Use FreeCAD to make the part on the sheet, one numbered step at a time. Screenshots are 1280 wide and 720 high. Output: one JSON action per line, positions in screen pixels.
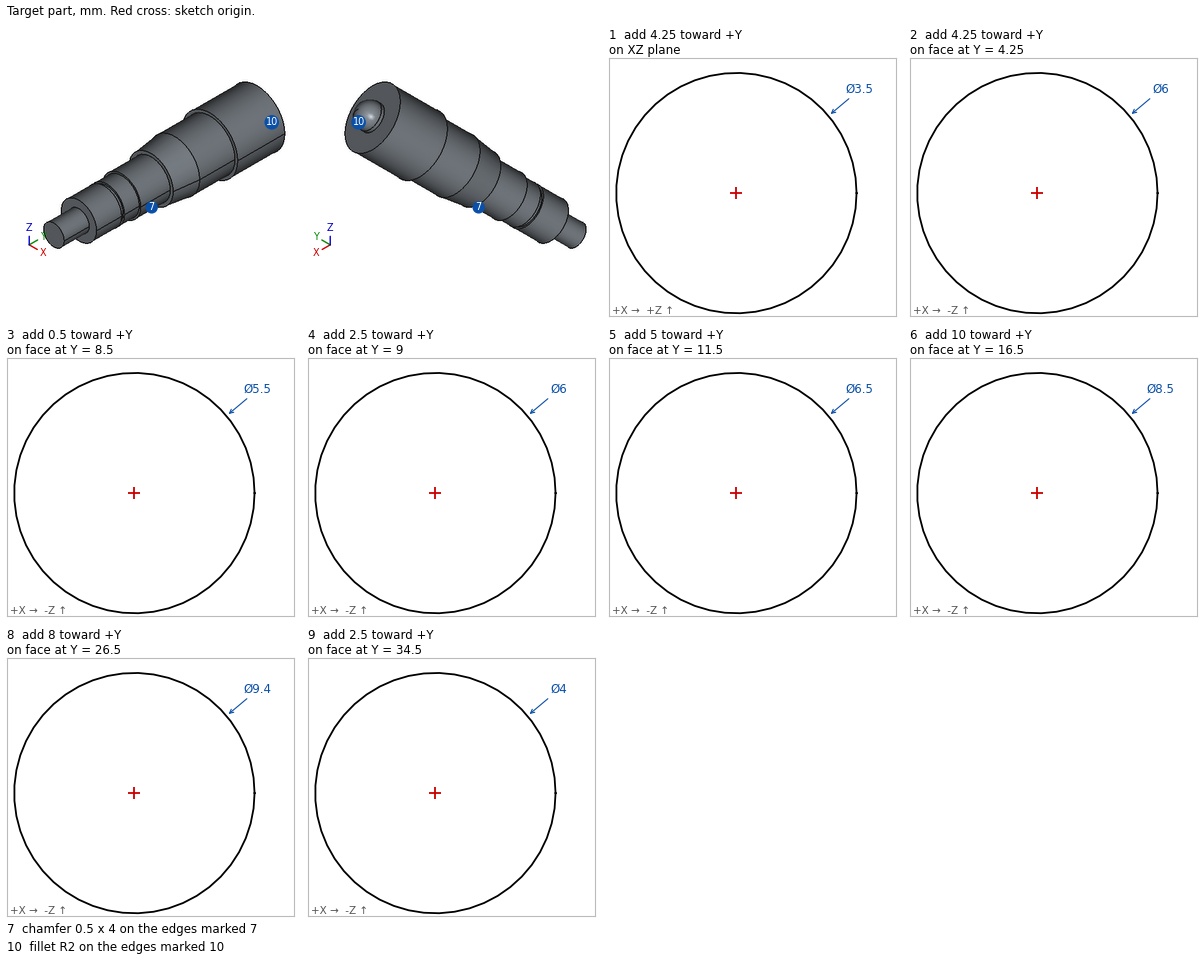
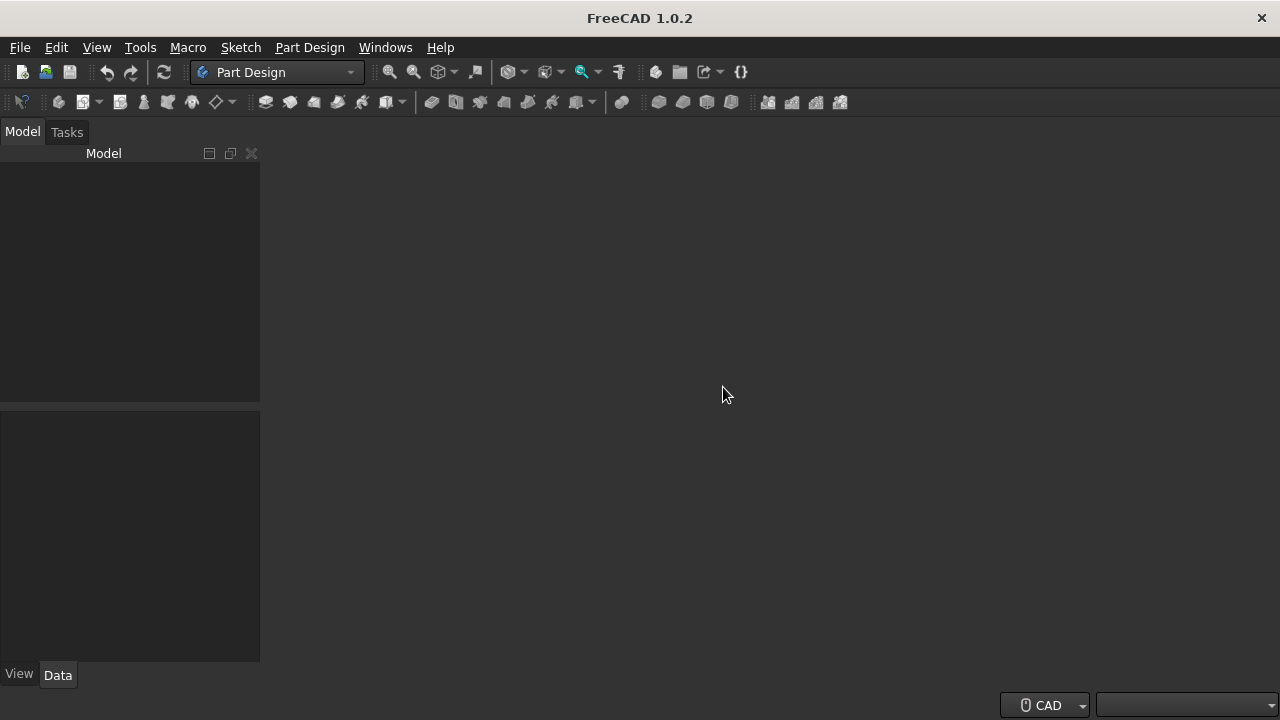
{"action": "key", "text": "ctrl+n"}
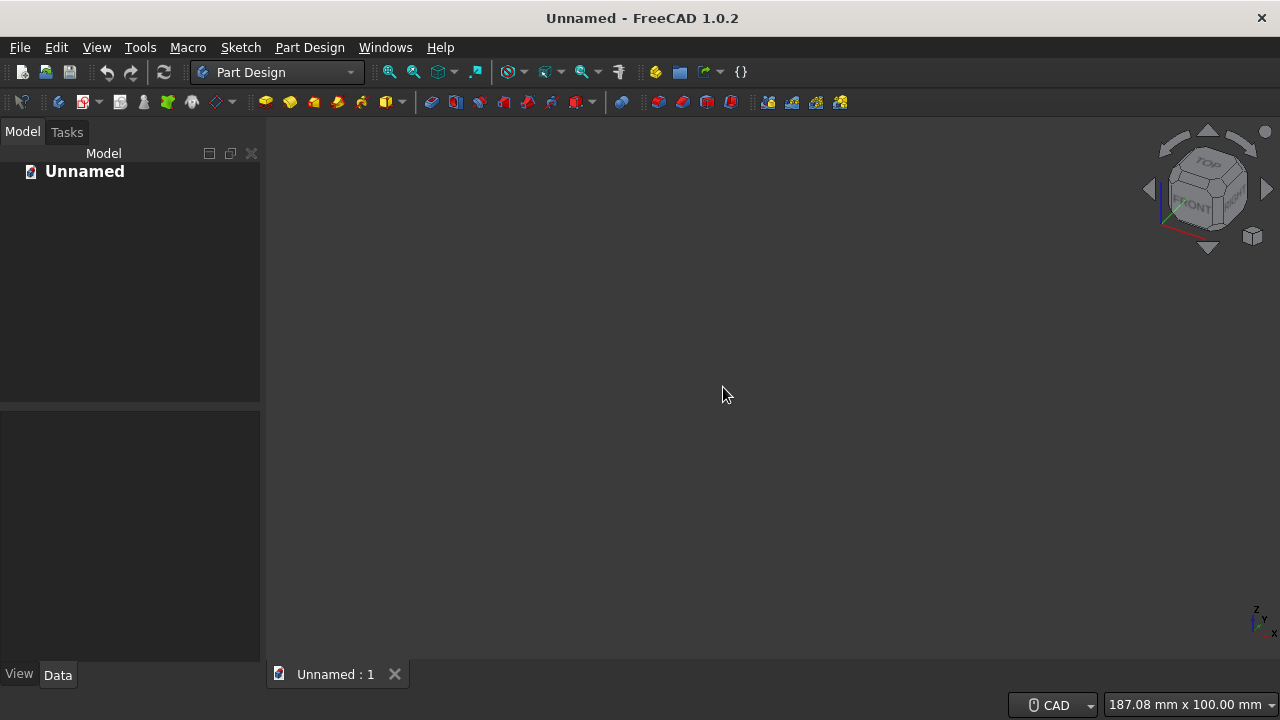
{"action": "left_click", "coordinate": [84, 102]}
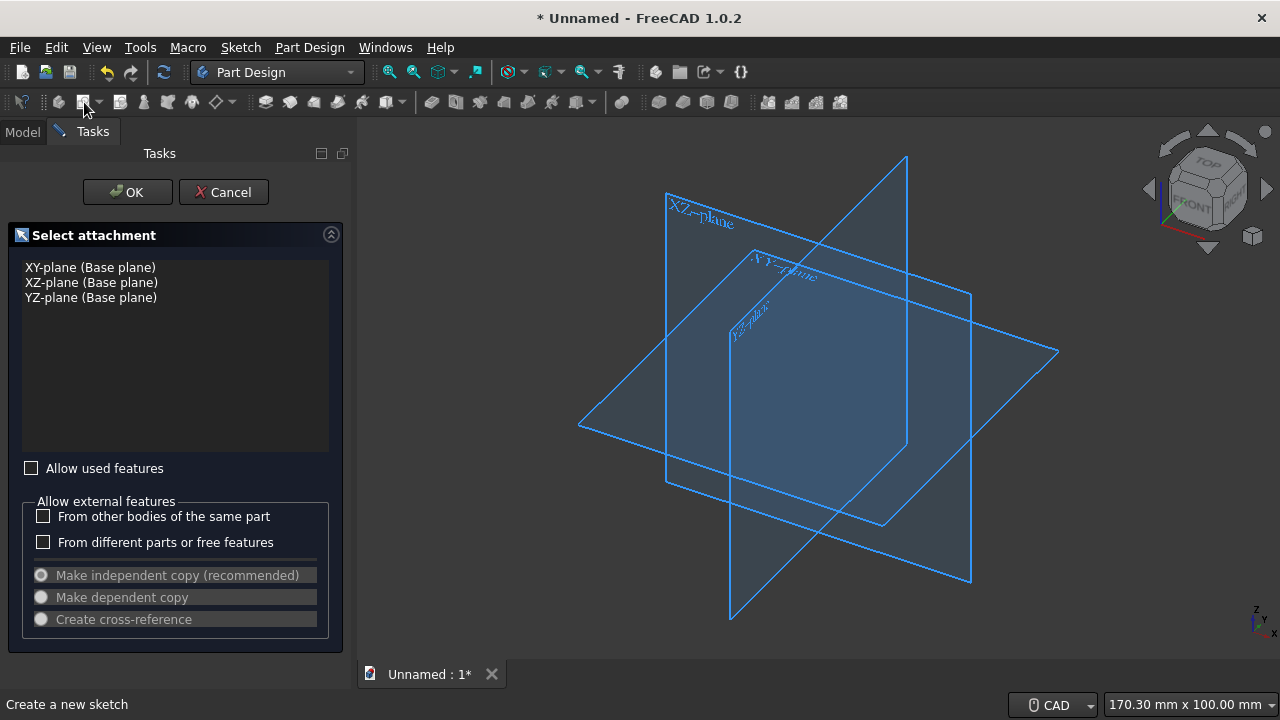
{"action": "left_click", "coordinate": [82, 282]}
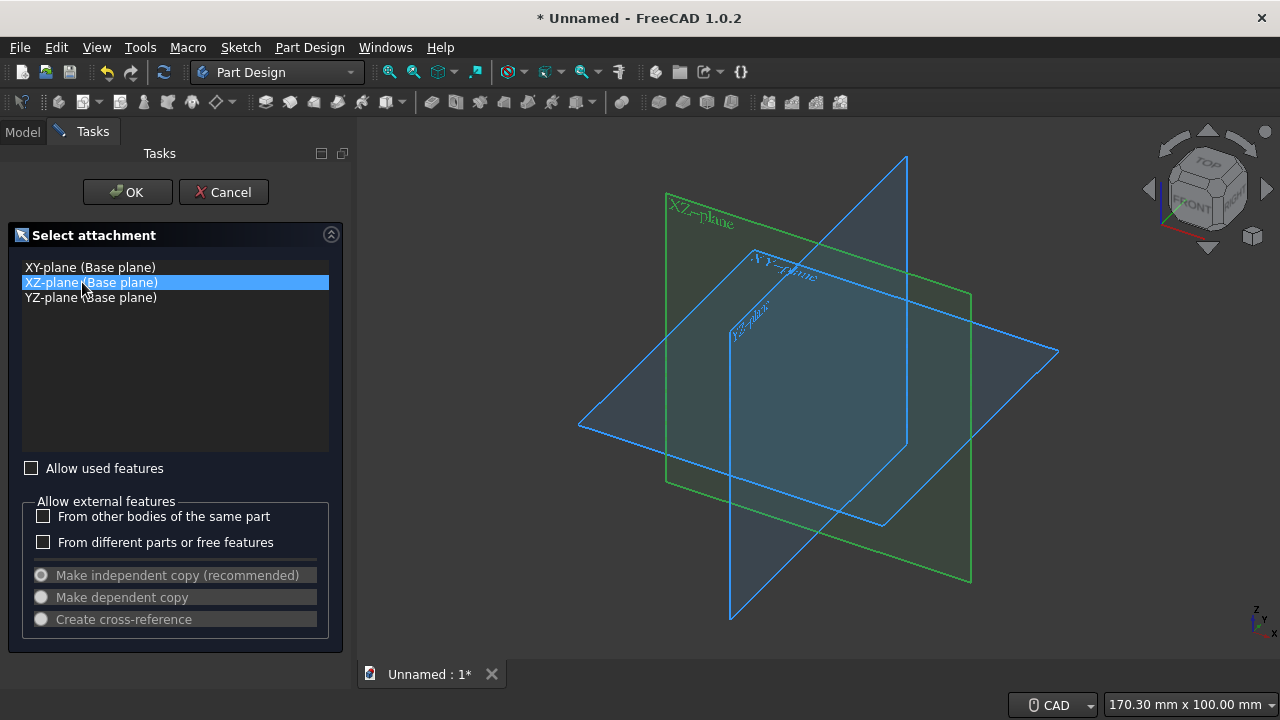
{"action": "left_click", "coordinate": [128, 192]}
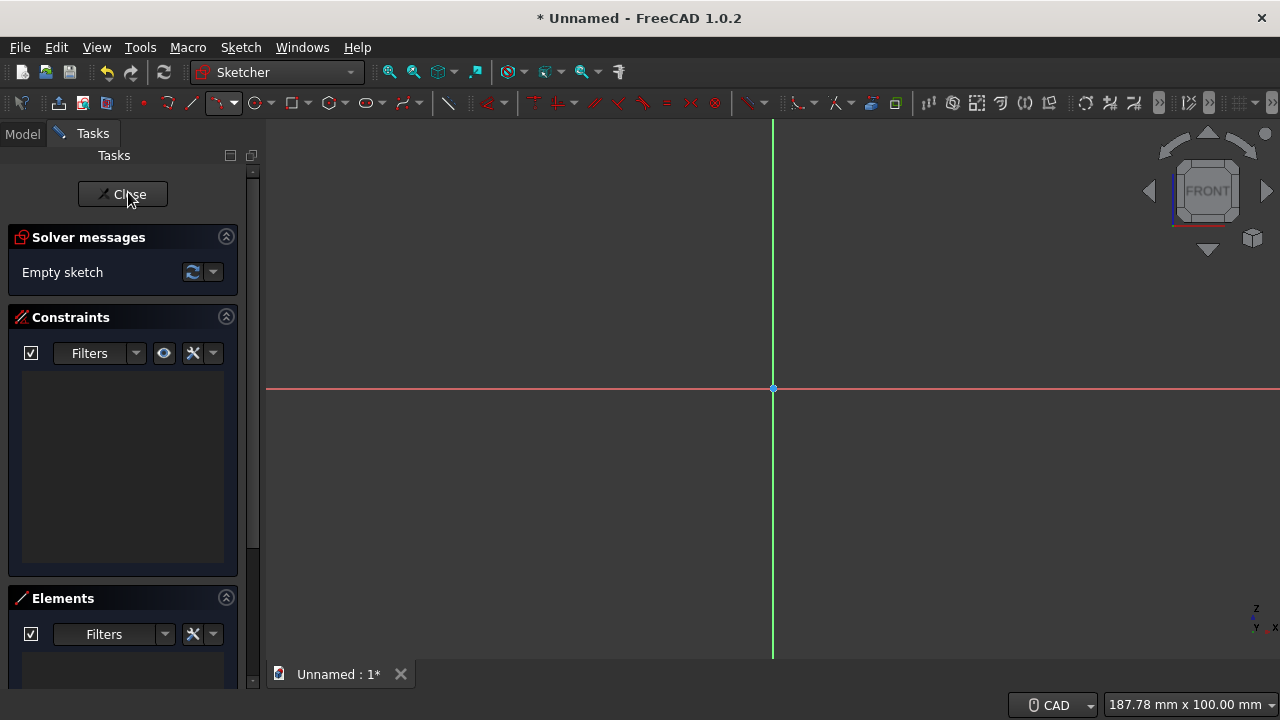
{"action": "scroll", "coordinate": [777, 389], "scroll_direction": "up", "scroll_amount": 14}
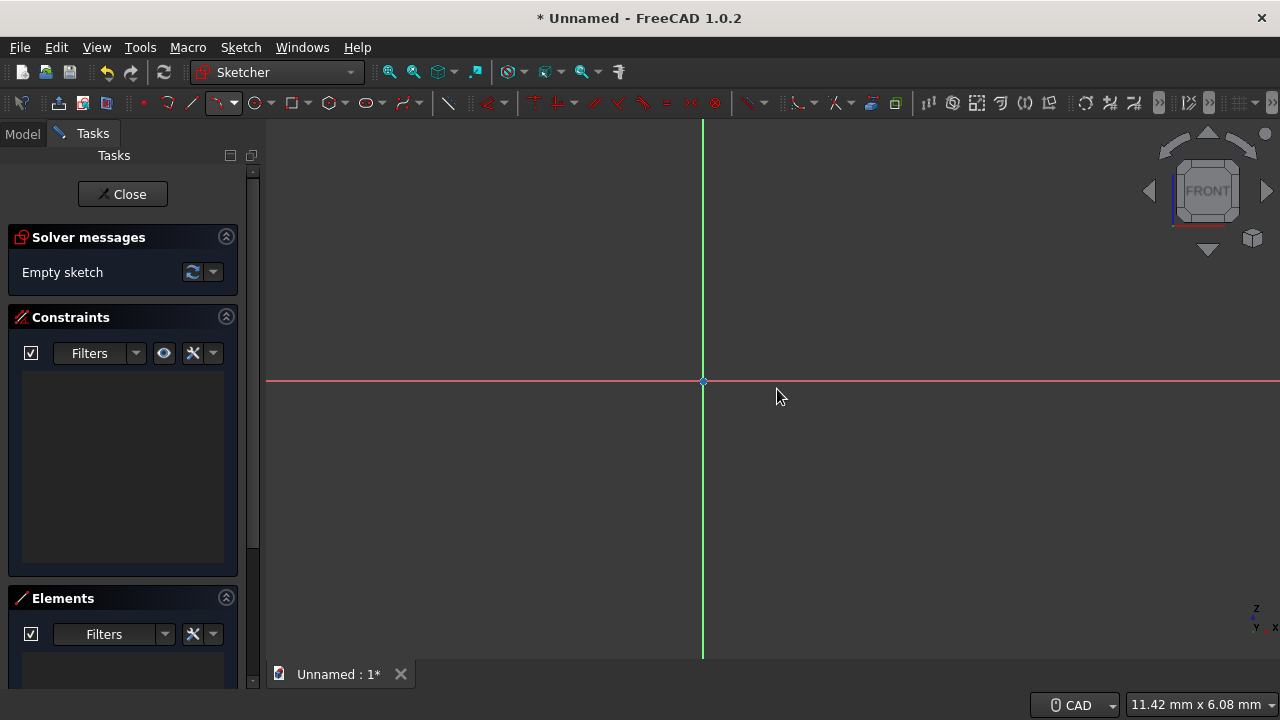
{"action": "key", "text": "g c"}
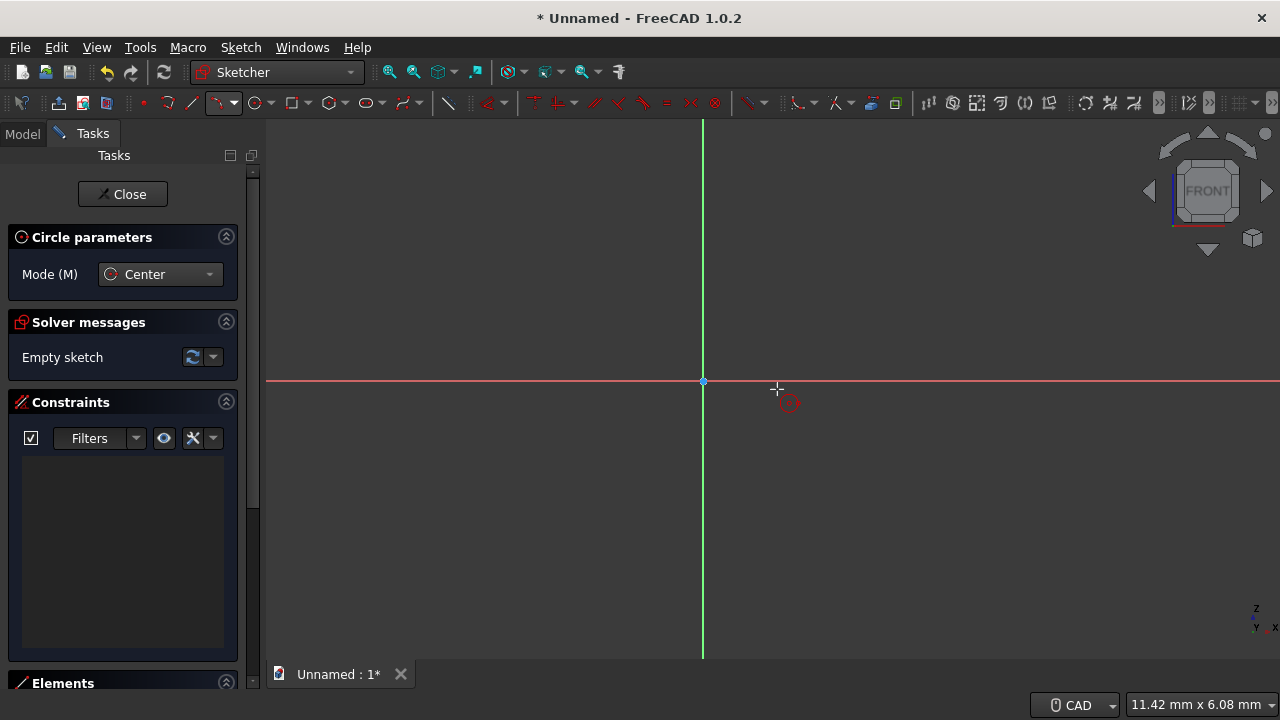
{"action": "left_click", "coordinate": [703, 381]}
{"action": "mouse_move", "coordinate": [813, 271]}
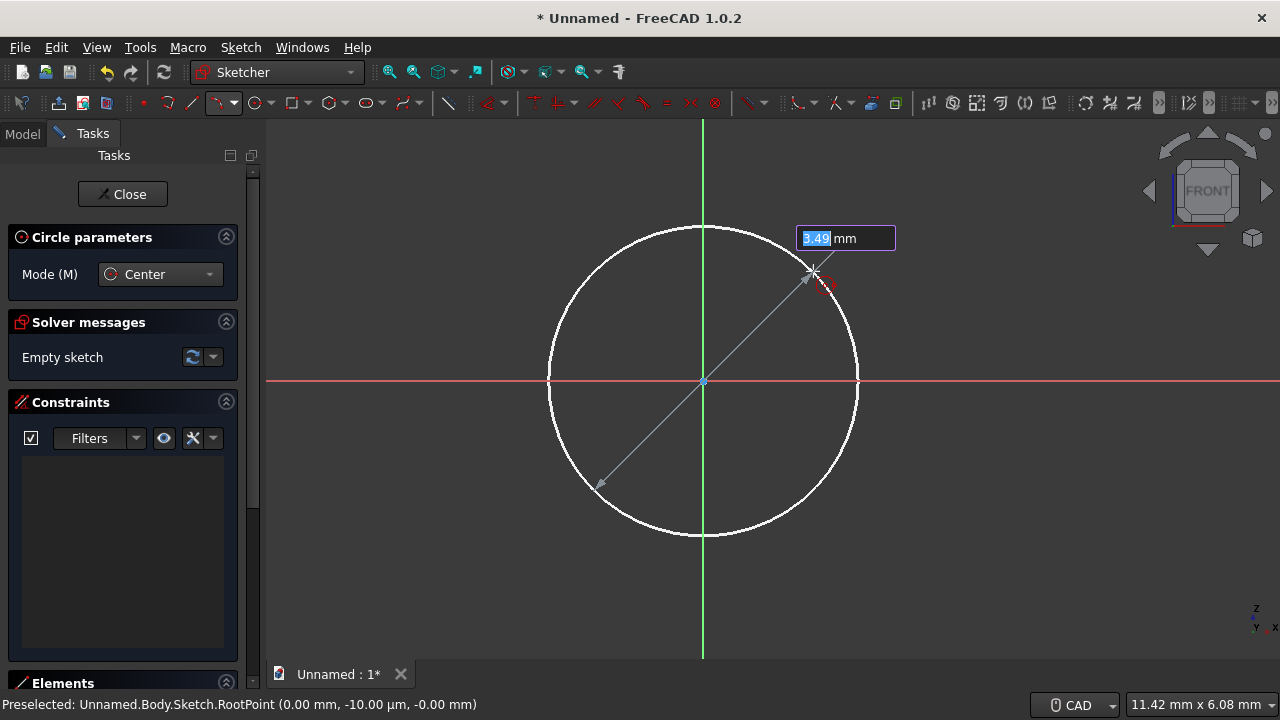
{"action": "type", "text": "3.5"}
{"action": "key", "text": "Return"}
{"action": "key", "text": "Escape"}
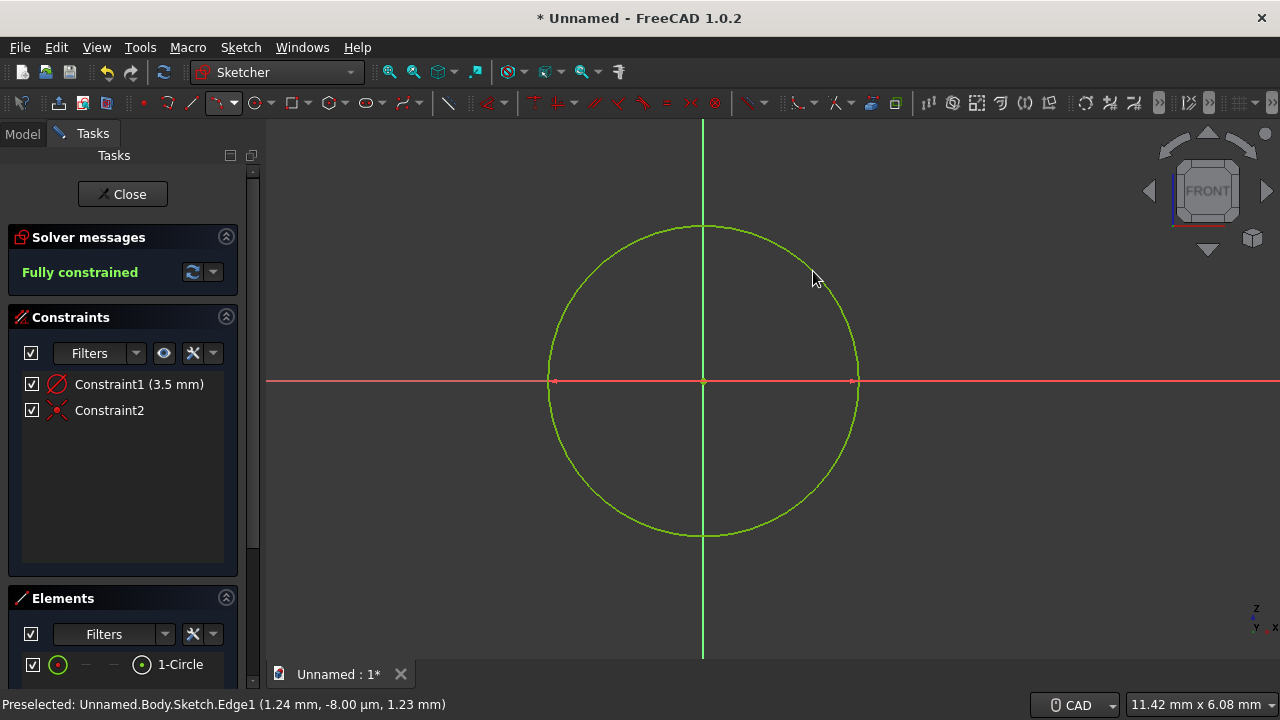
{"action": "left_click", "coordinate": [123, 194]}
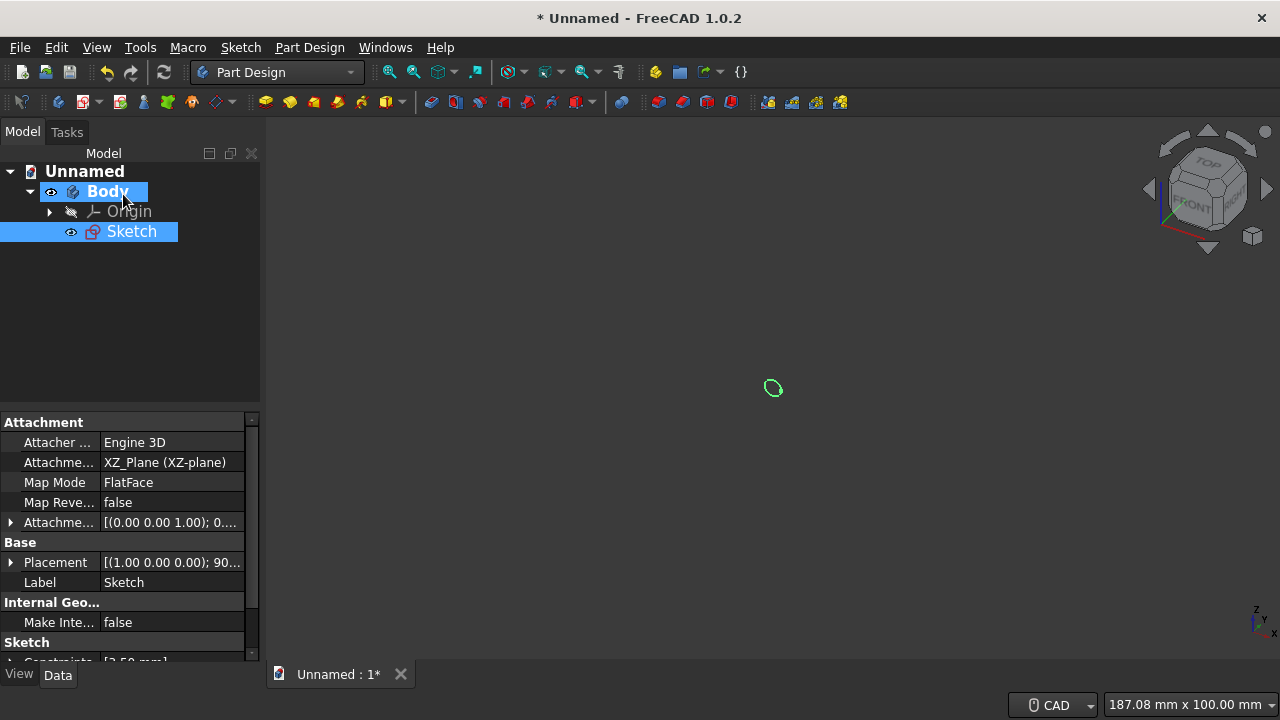
{"action": "left_click", "coordinate": [266, 102]}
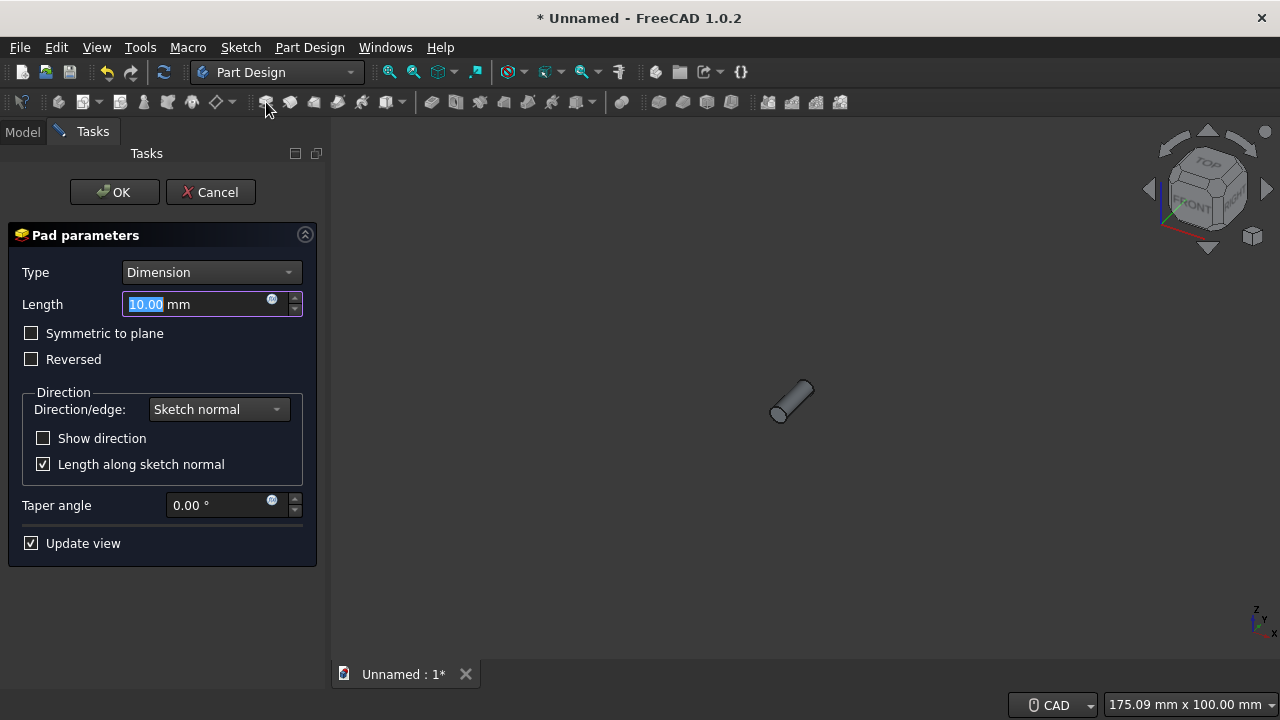
{"action": "type", "text": "4.25"}
{"action": "key", "text": "Tab"}